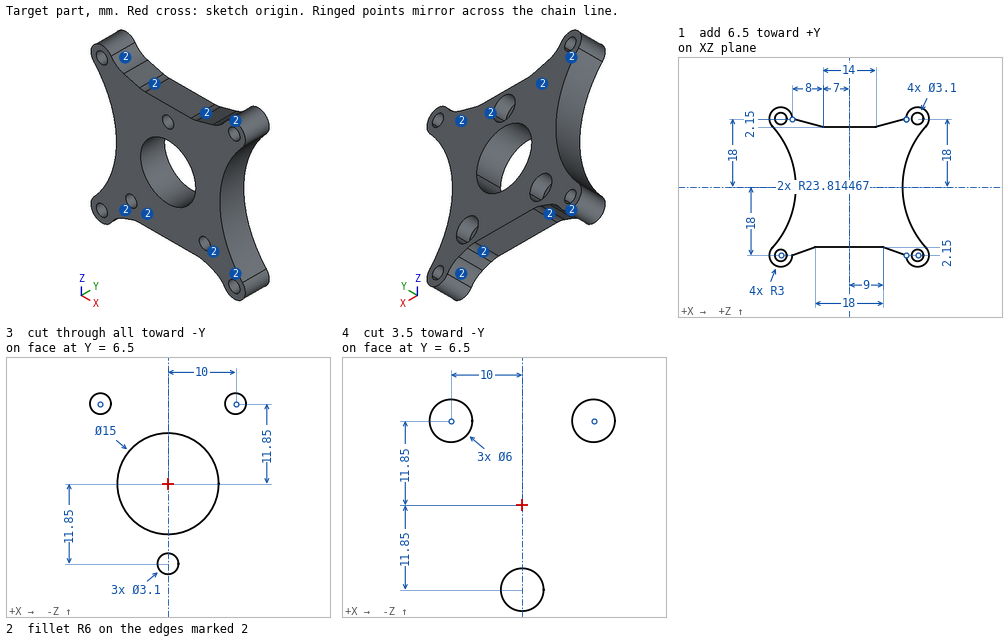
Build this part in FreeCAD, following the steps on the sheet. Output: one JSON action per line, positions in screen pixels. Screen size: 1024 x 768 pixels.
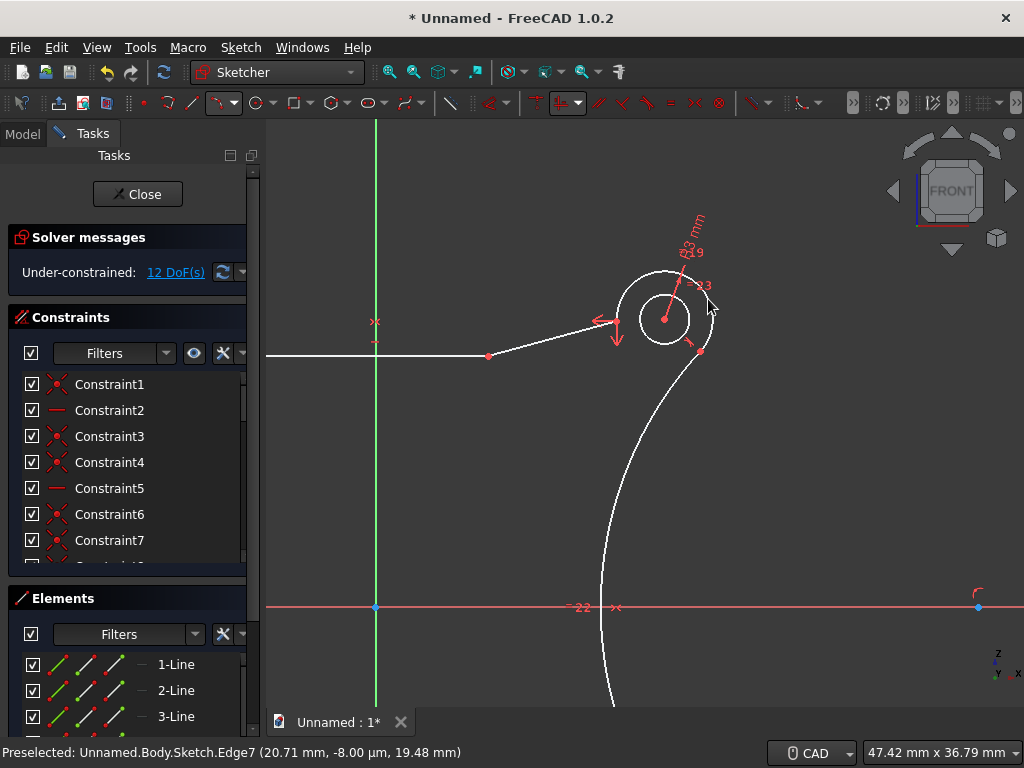
{"action": "left_click", "coordinate": [617, 497]}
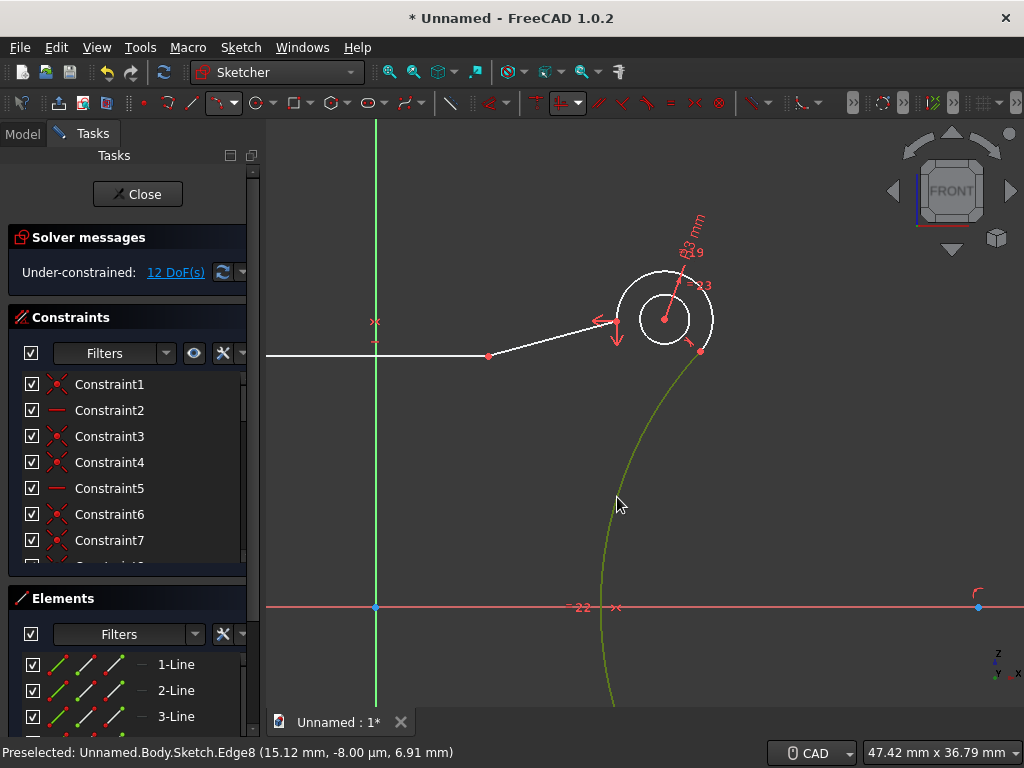
{"action": "left_click", "coordinate": [508, 104]}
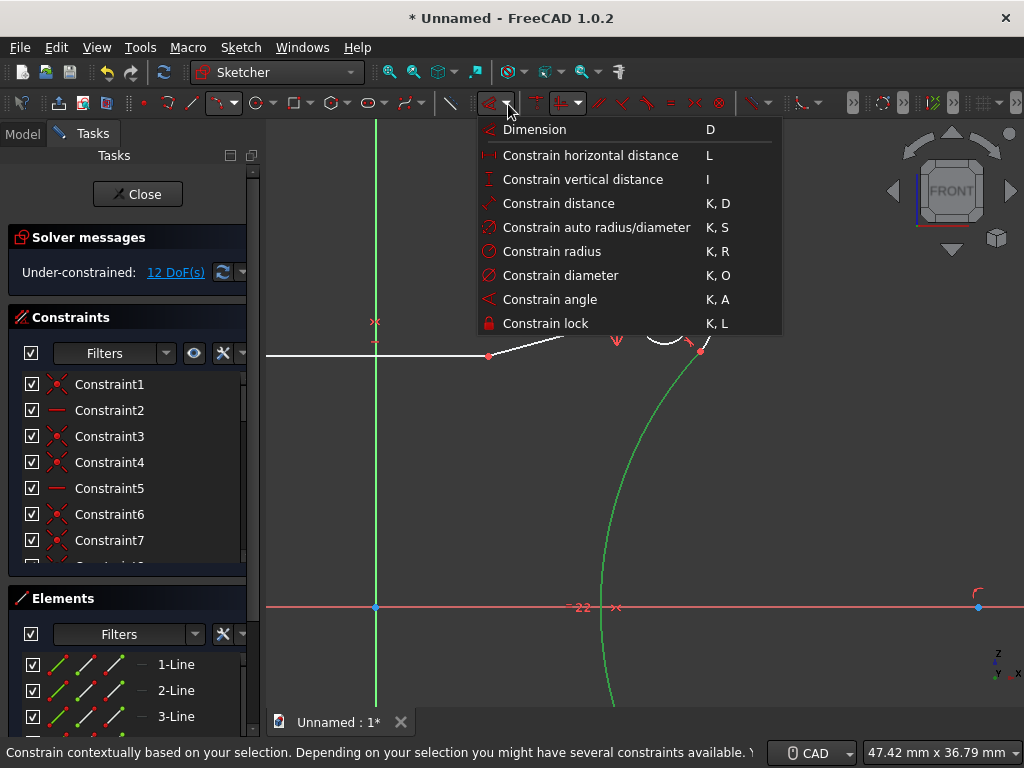
{"action": "left_click", "coordinate": [630, 251]}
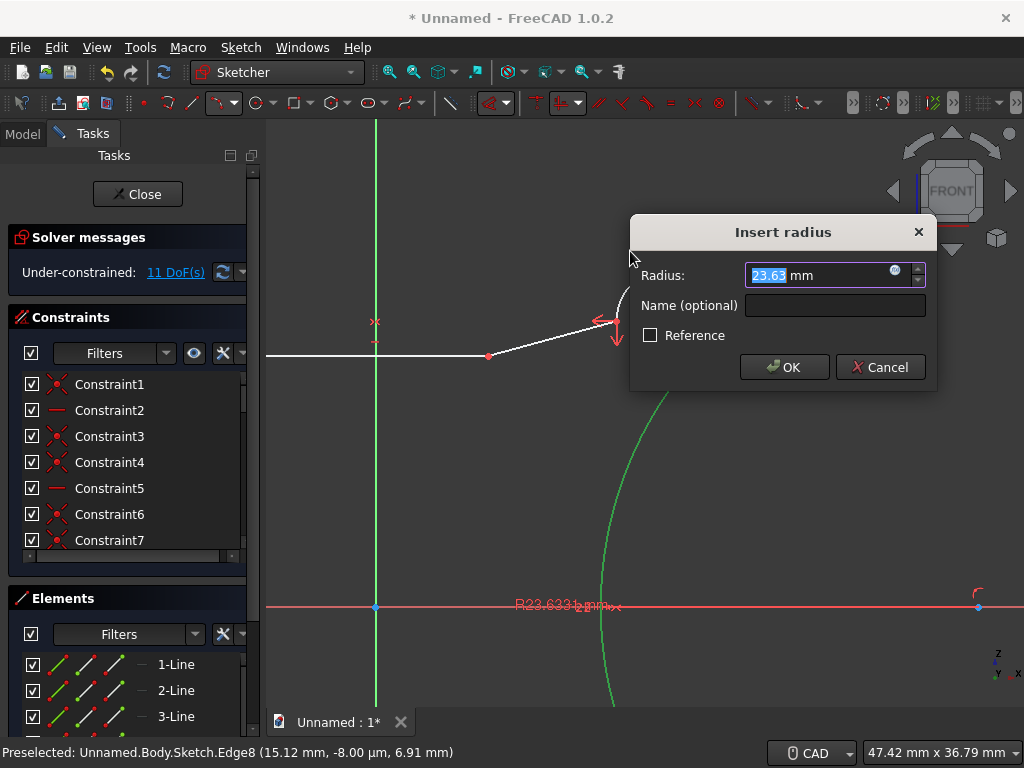
{"action": "type", "text": "23.814467"}
{"action": "key", "text": "Return"}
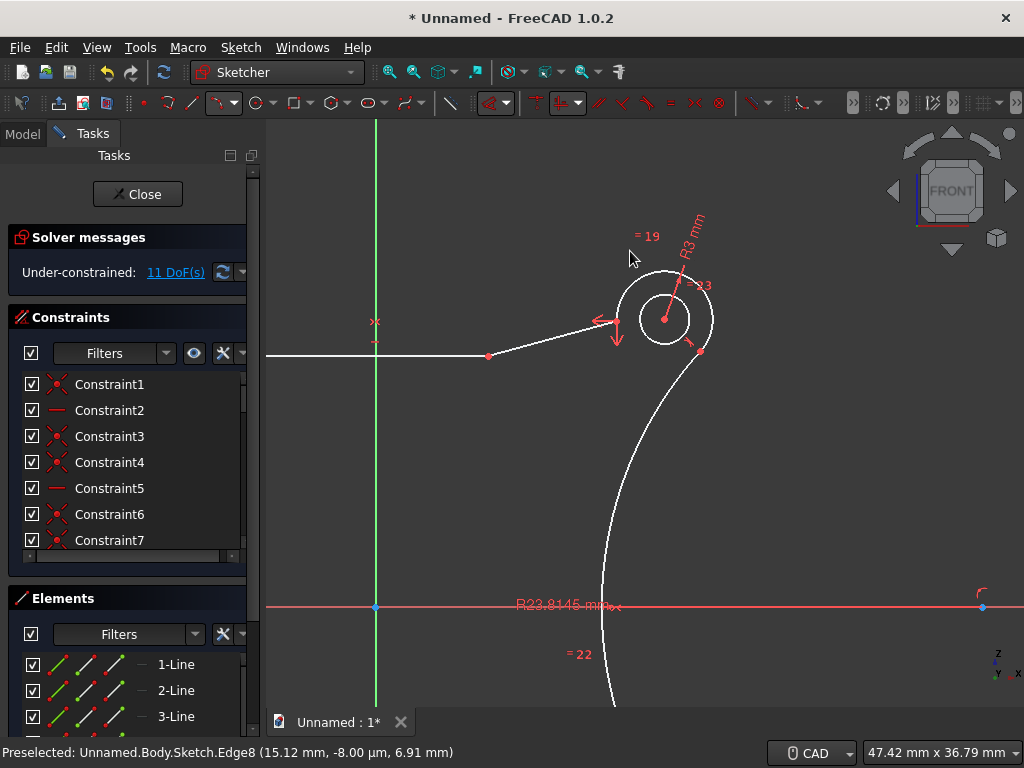
{"action": "left_click", "coordinate": [682, 302]}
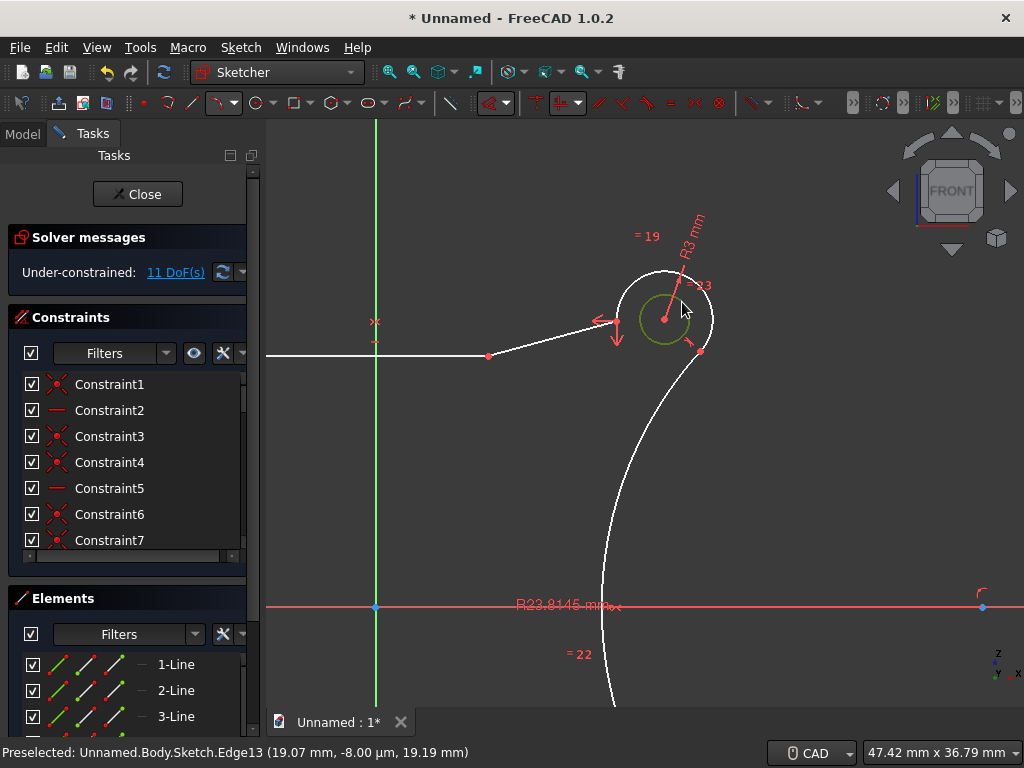
{"action": "left_click", "coordinate": [508, 104]}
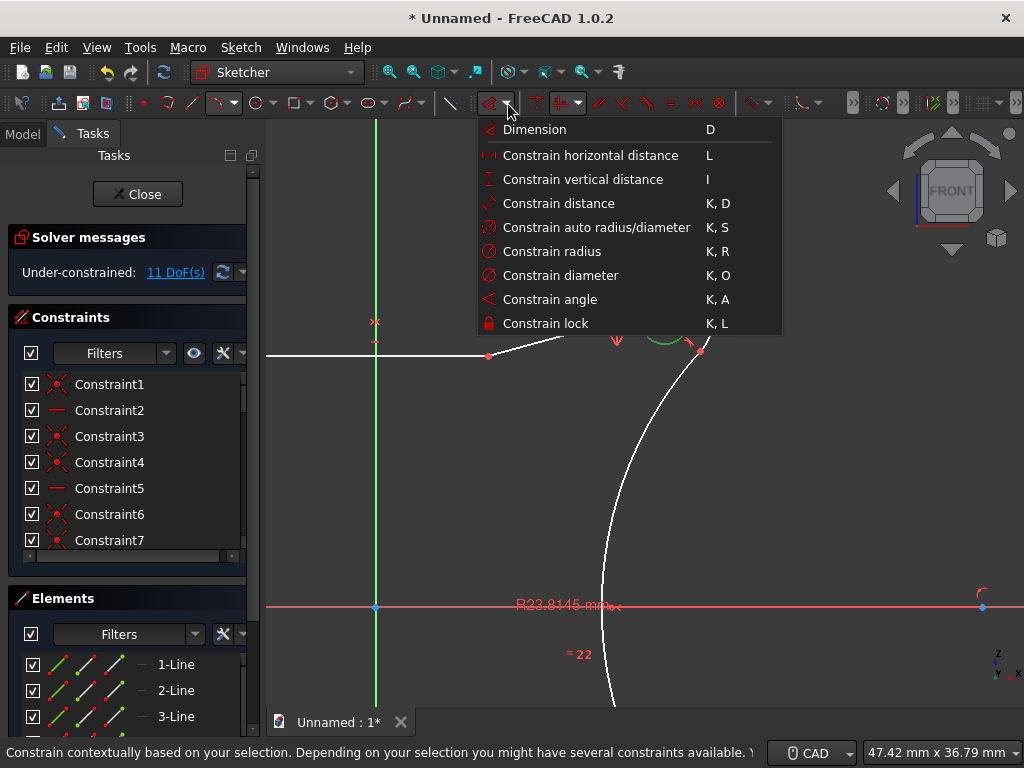
{"action": "left_click", "coordinate": [630, 275]}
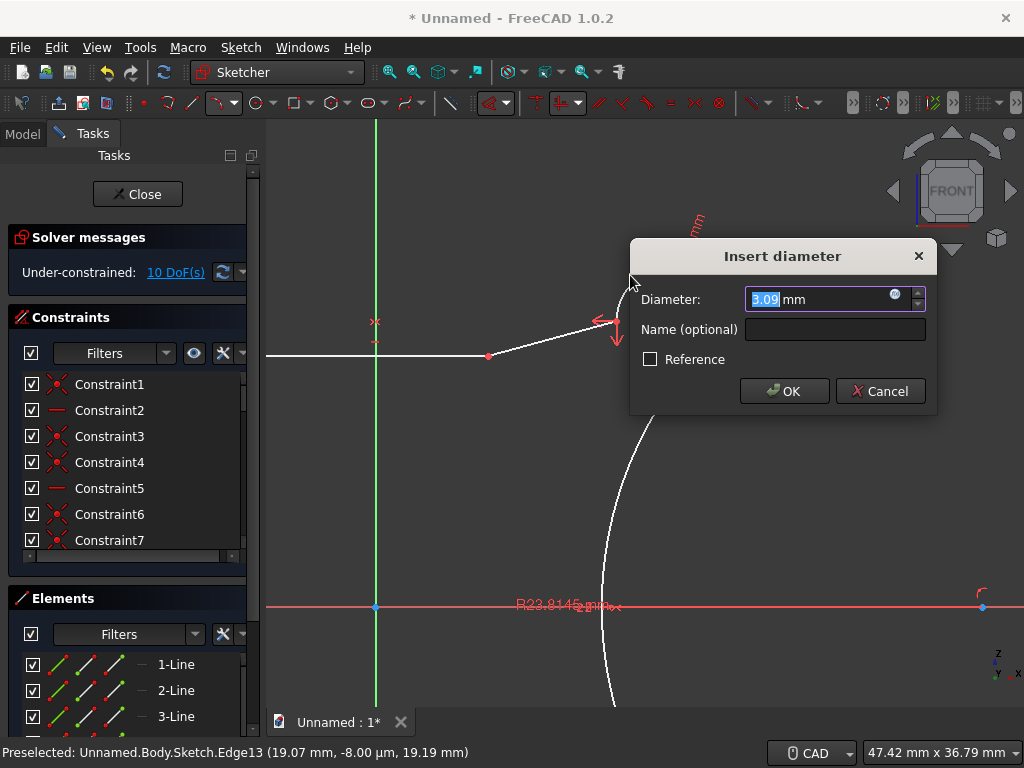
{"action": "type", "text": "3.1"}
{"action": "key", "text": "Return"}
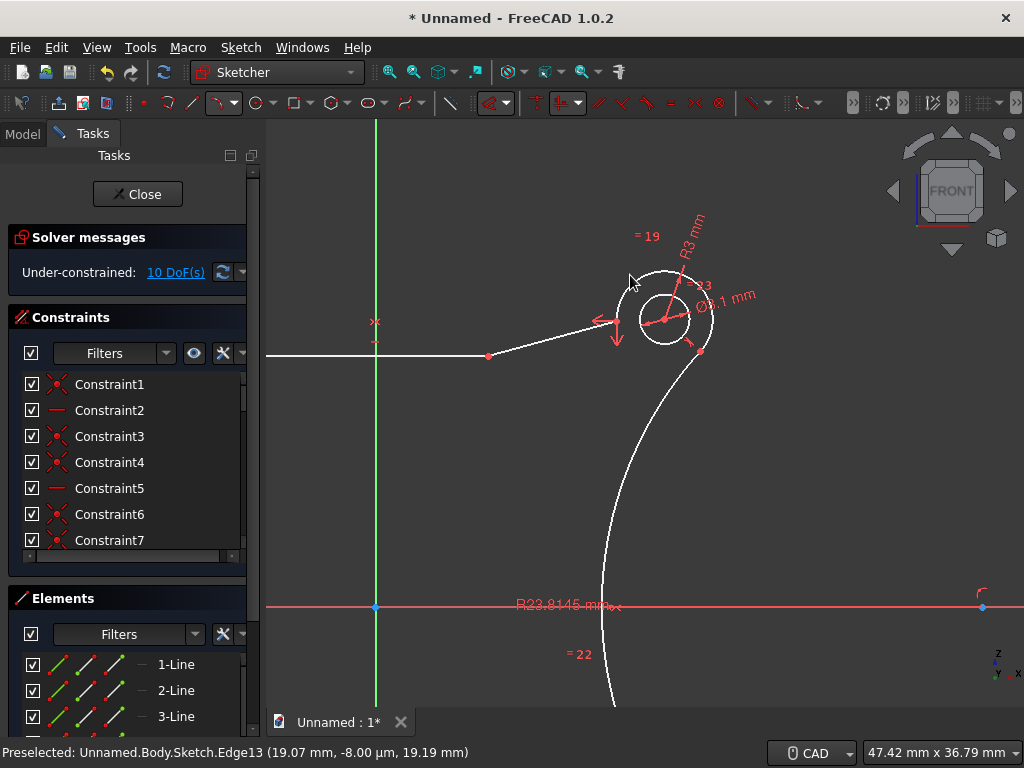
{"action": "left_click", "coordinate": [331, 356]}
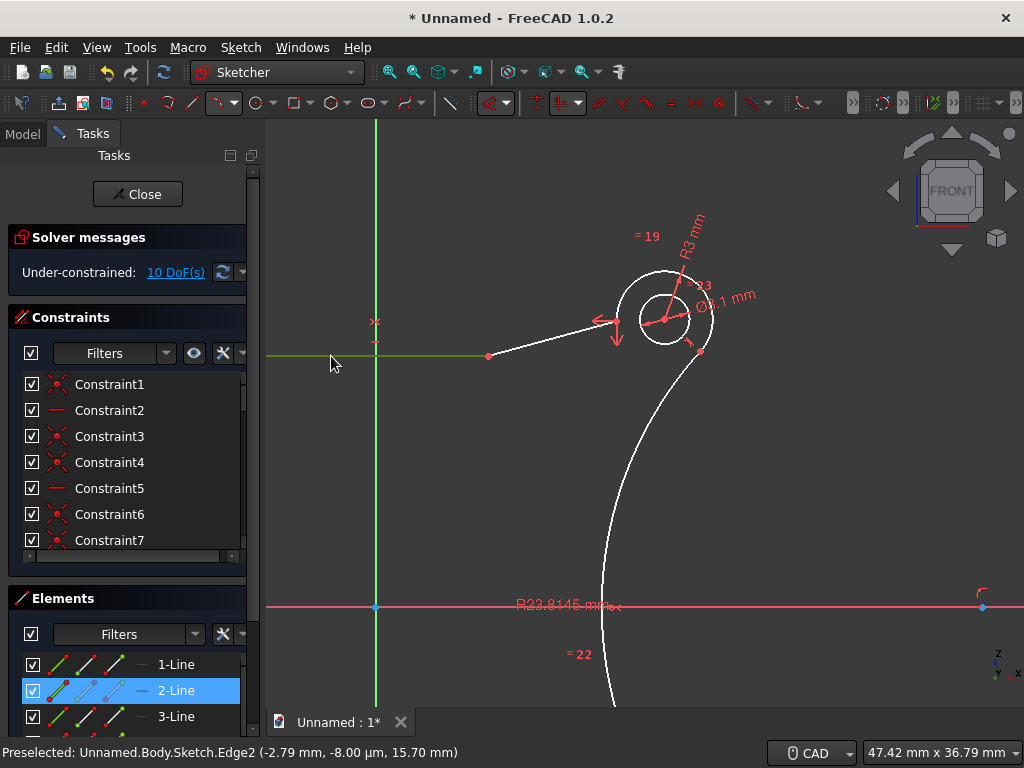
{"action": "left_click", "coordinate": [508, 104]}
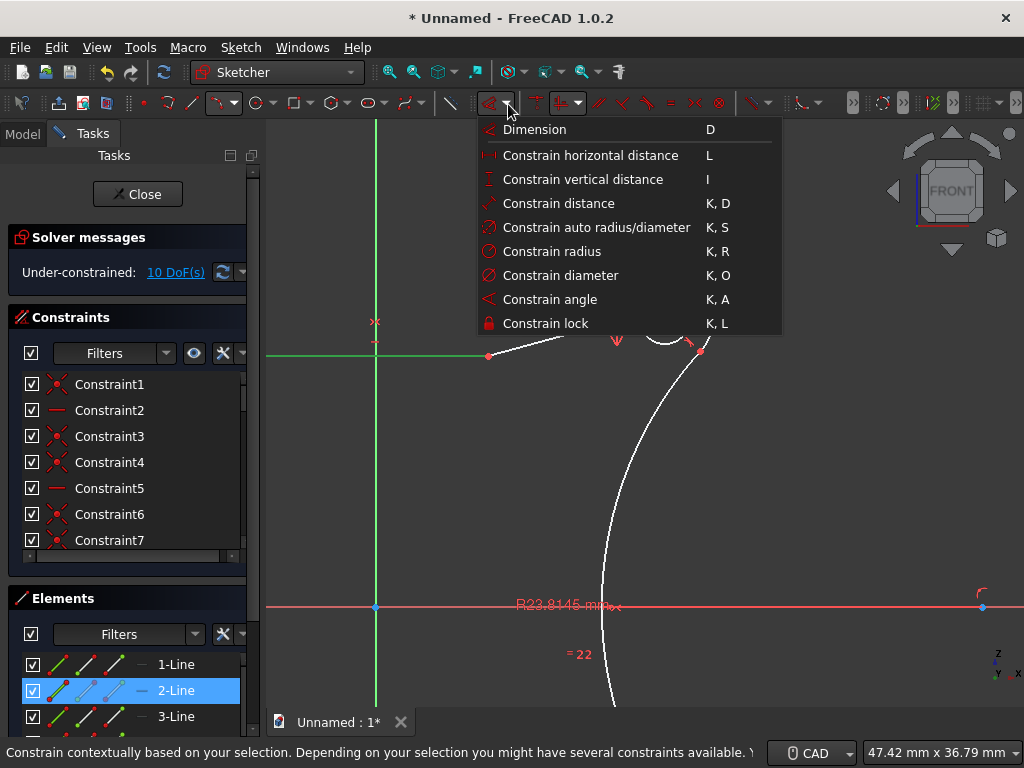
{"action": "left_click", "coordinate": [630, 155]}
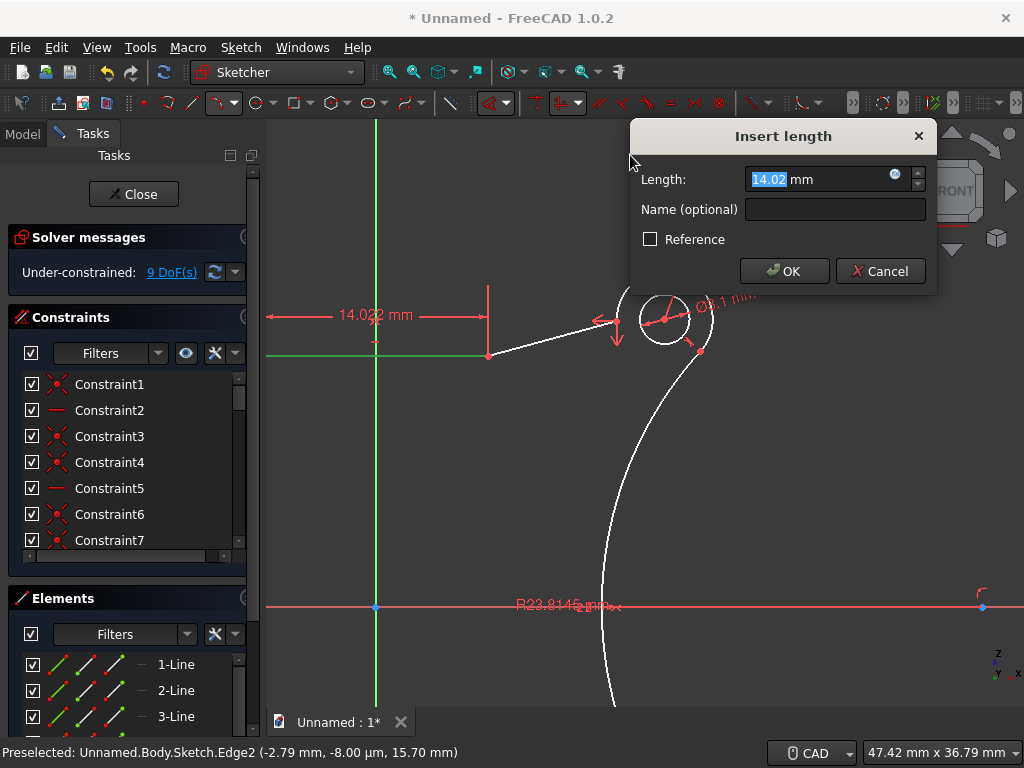
{"action": "type", "text": "14"}
{"action": "key", "text": "Return"}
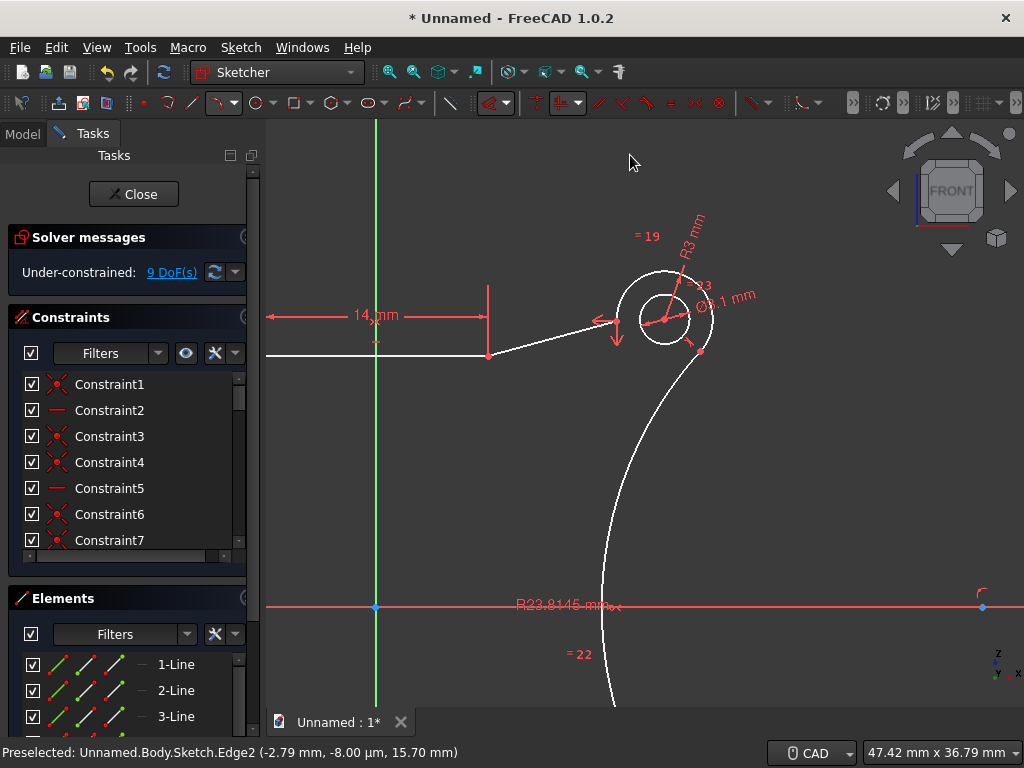
{"action": "scroll", "coordinate": [821, 177], "scroll_direction": "down", "scroll_amount": 3}